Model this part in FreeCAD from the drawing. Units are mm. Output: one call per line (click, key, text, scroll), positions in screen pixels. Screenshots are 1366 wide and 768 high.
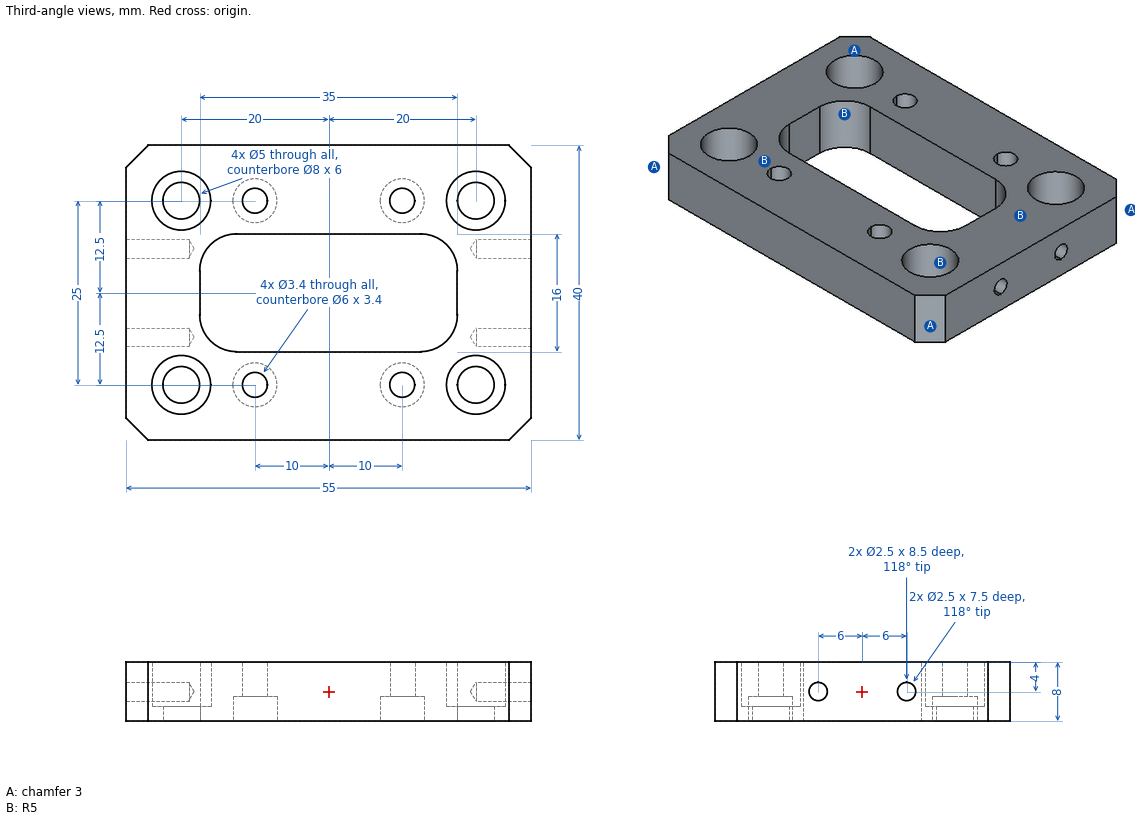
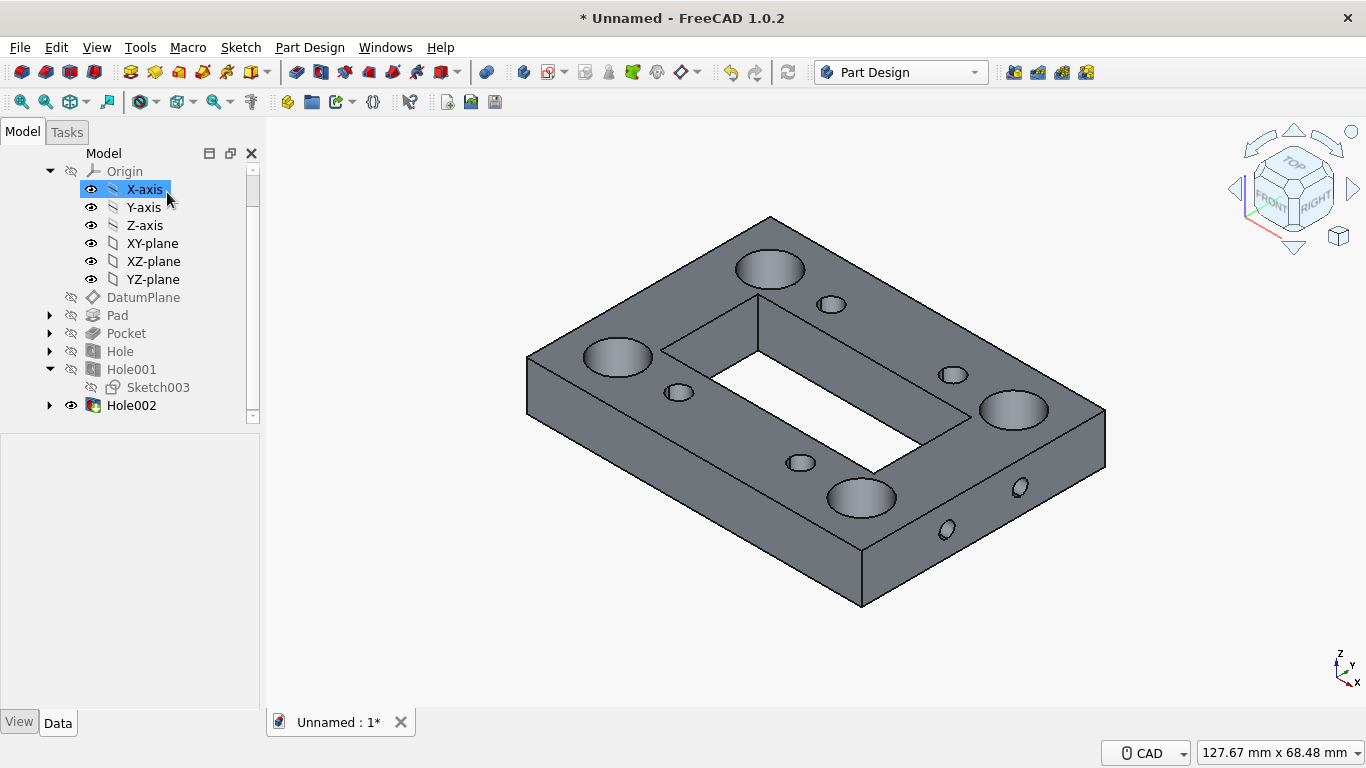
key(6)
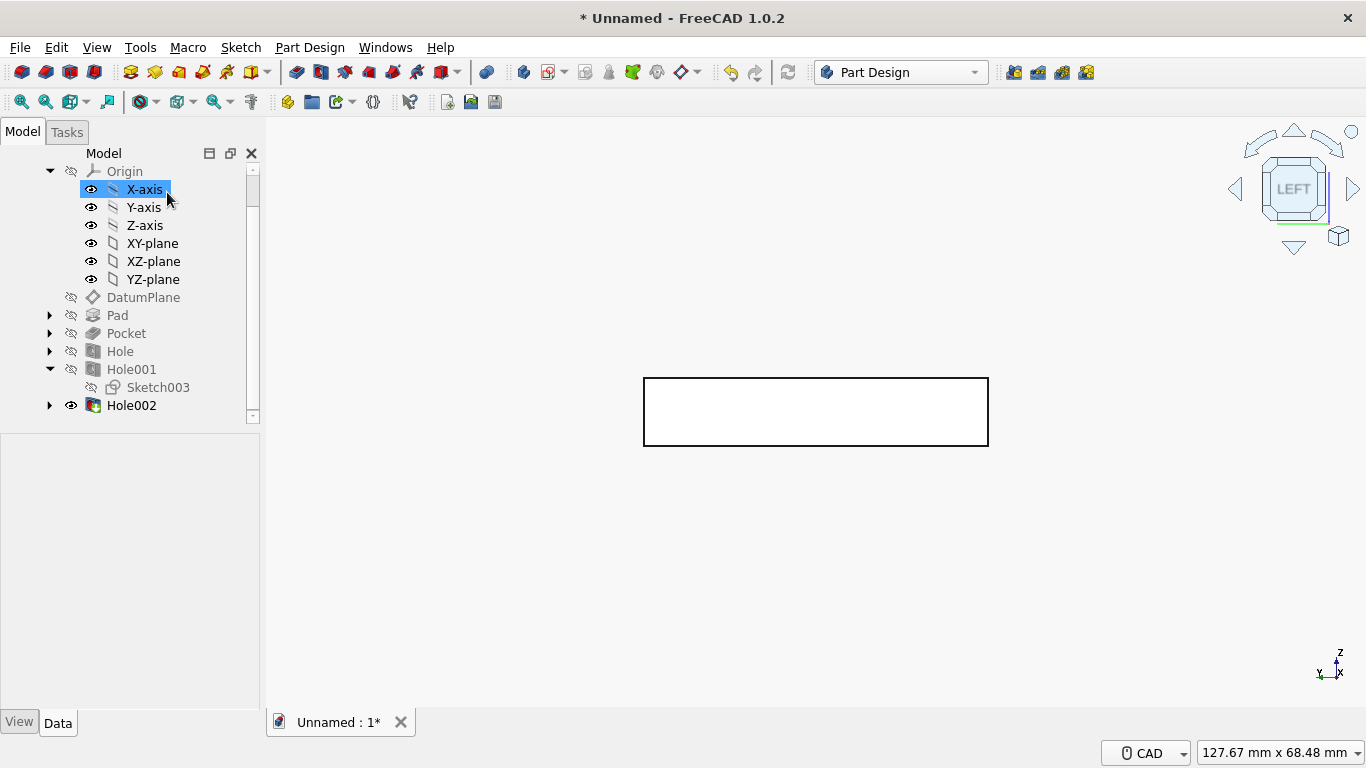
click(22, 102)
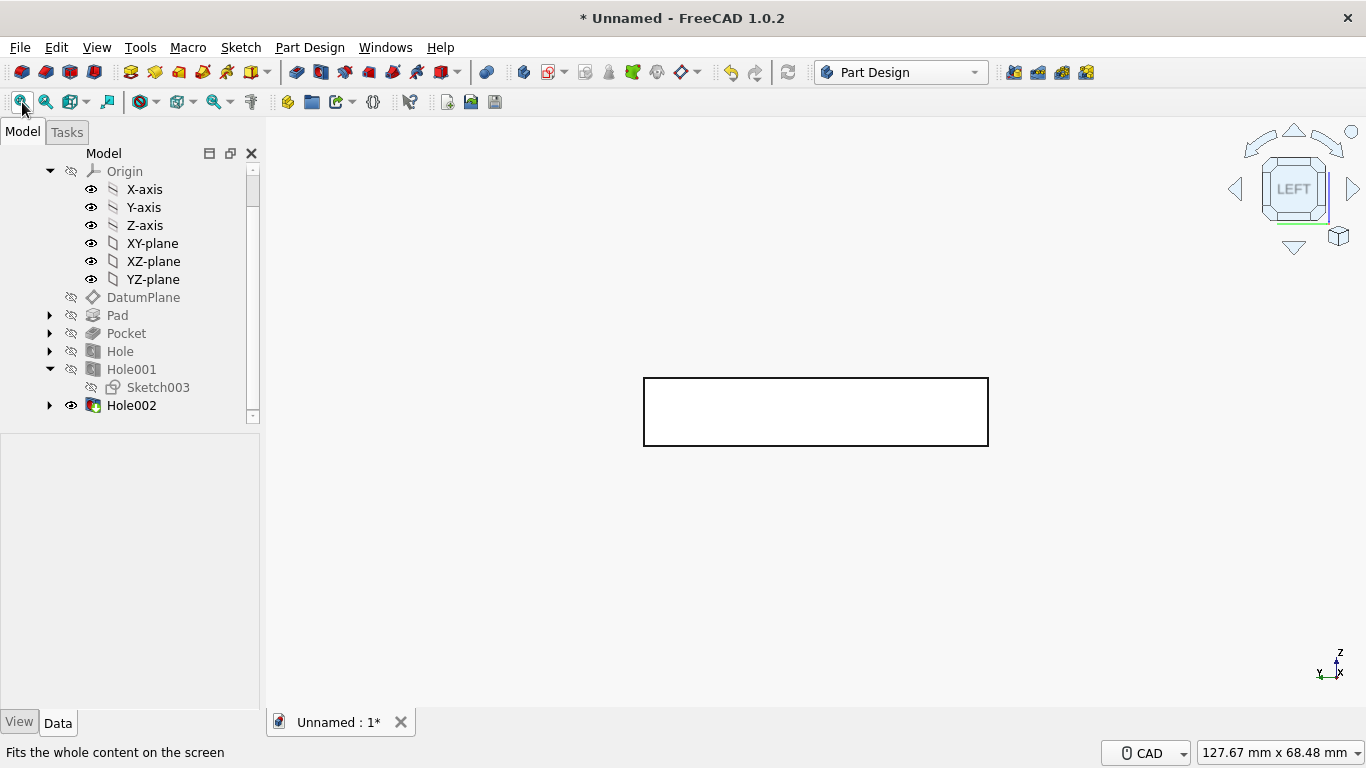
click(718, 411)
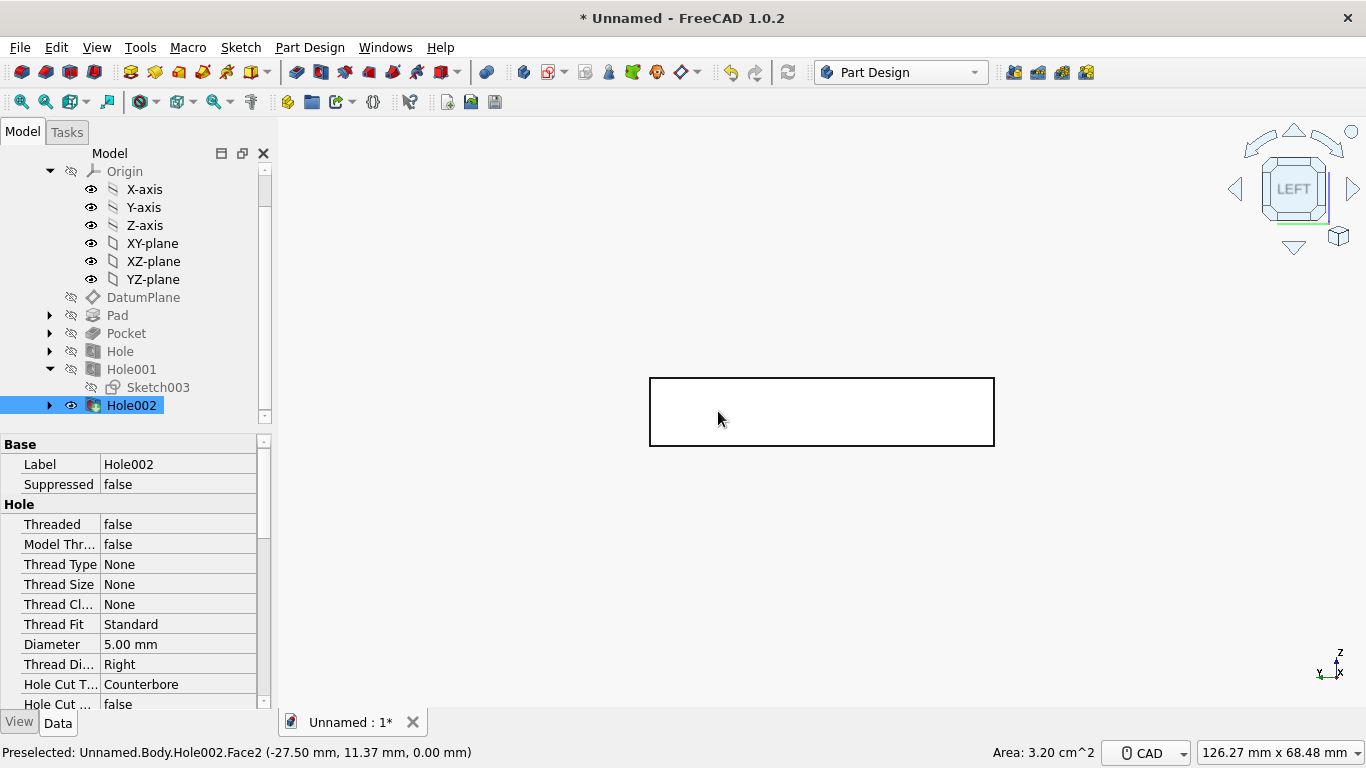
click(548, 72)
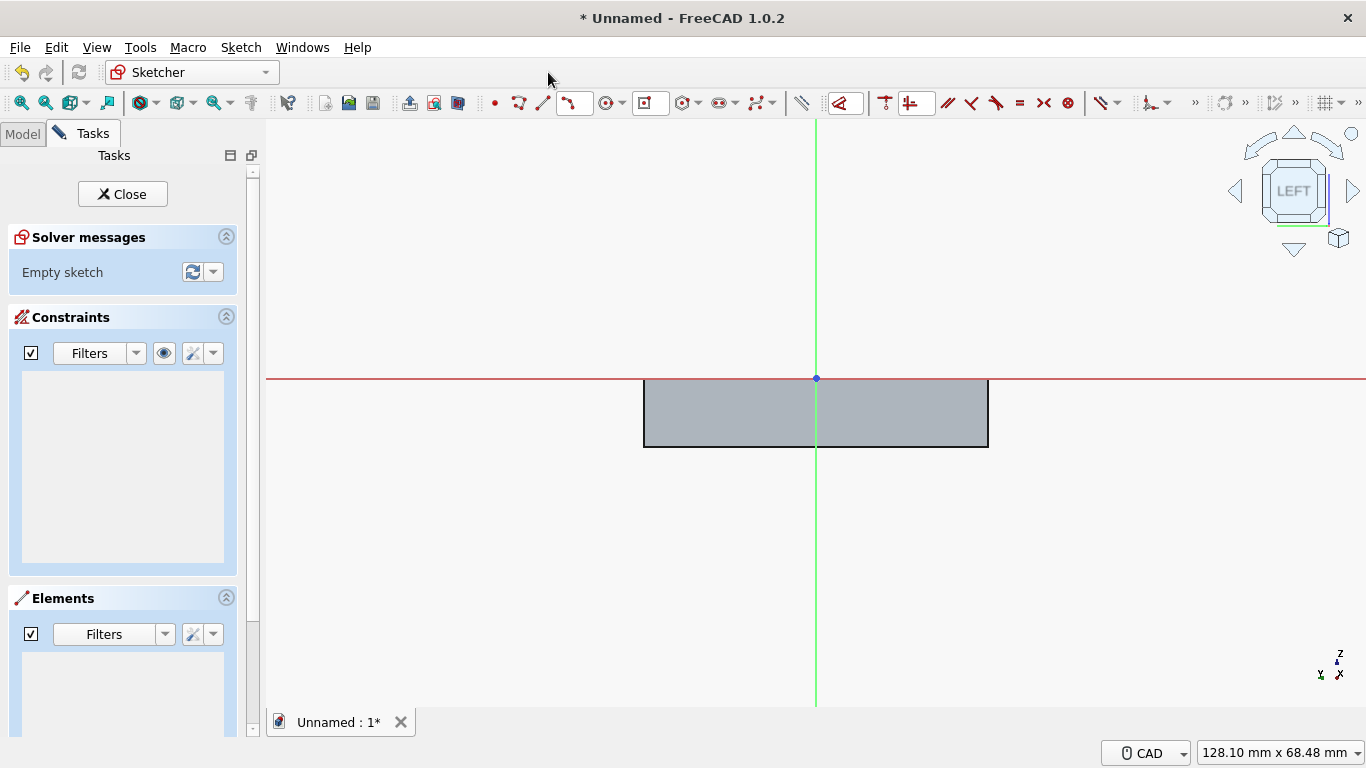
scroll(833, 398, up, 8)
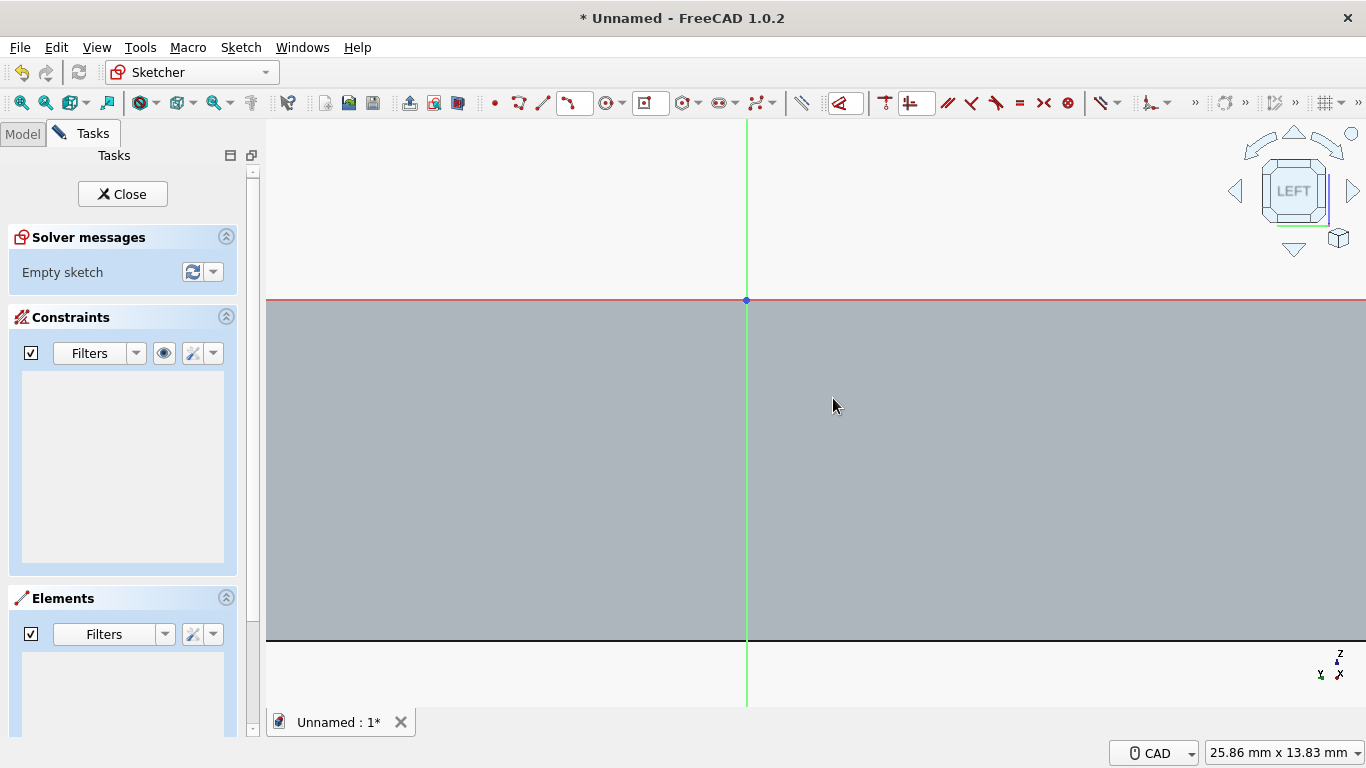
click(606, 104)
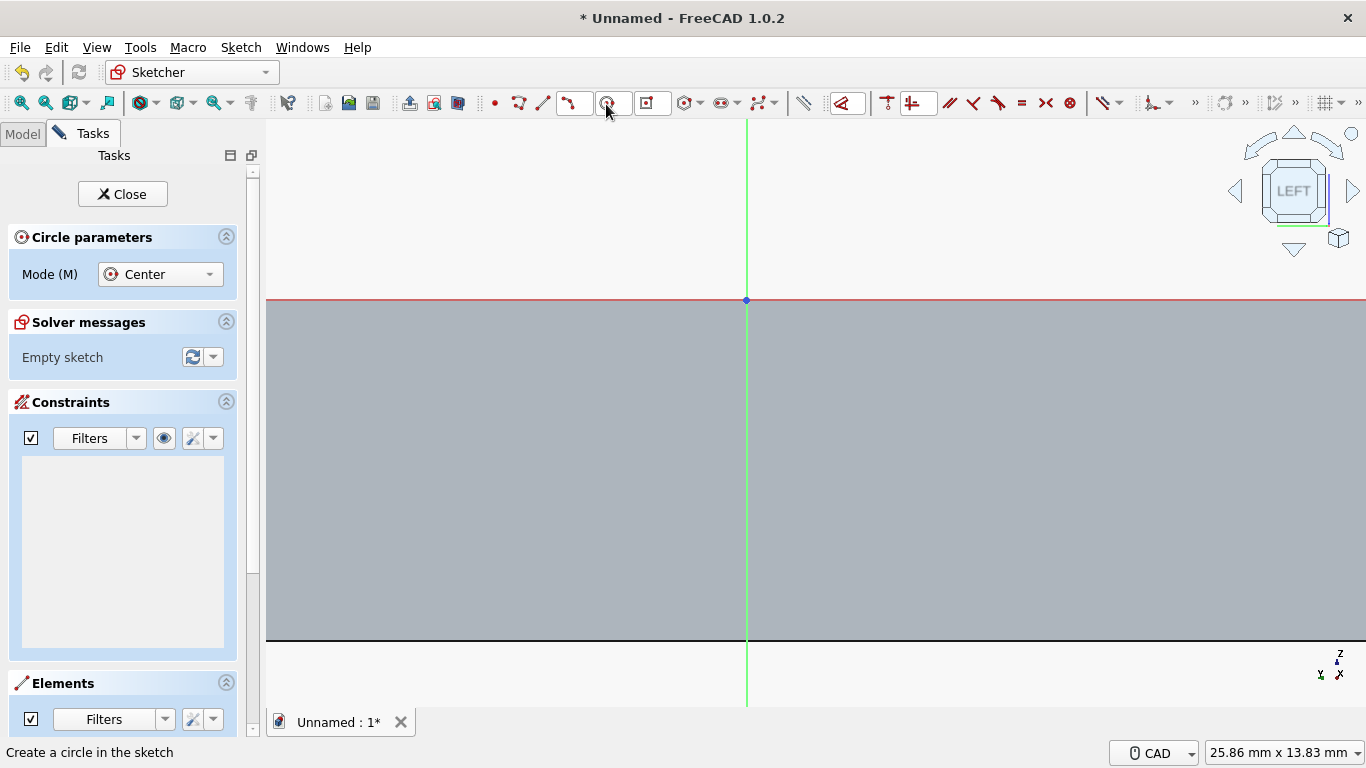
click(492, 470)
move(529, 433)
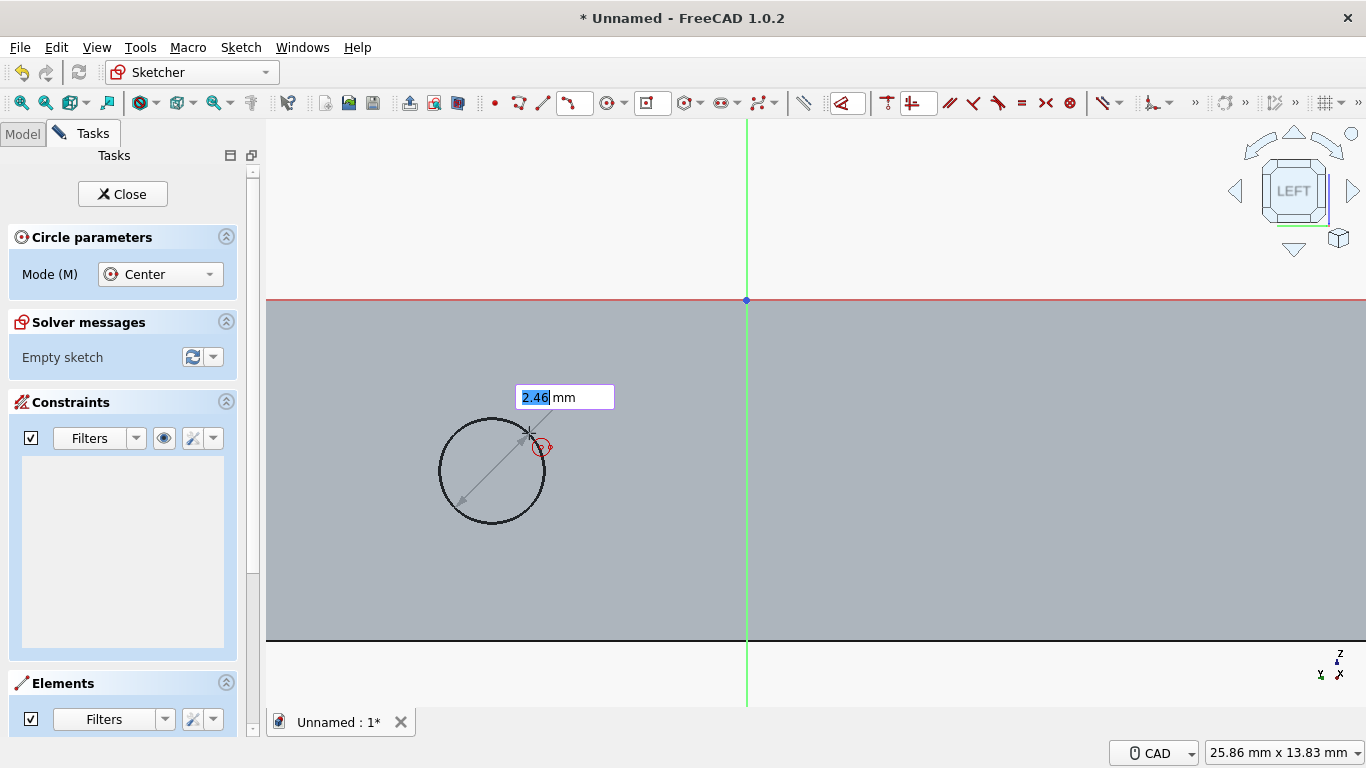
text(2.5)
key(Return)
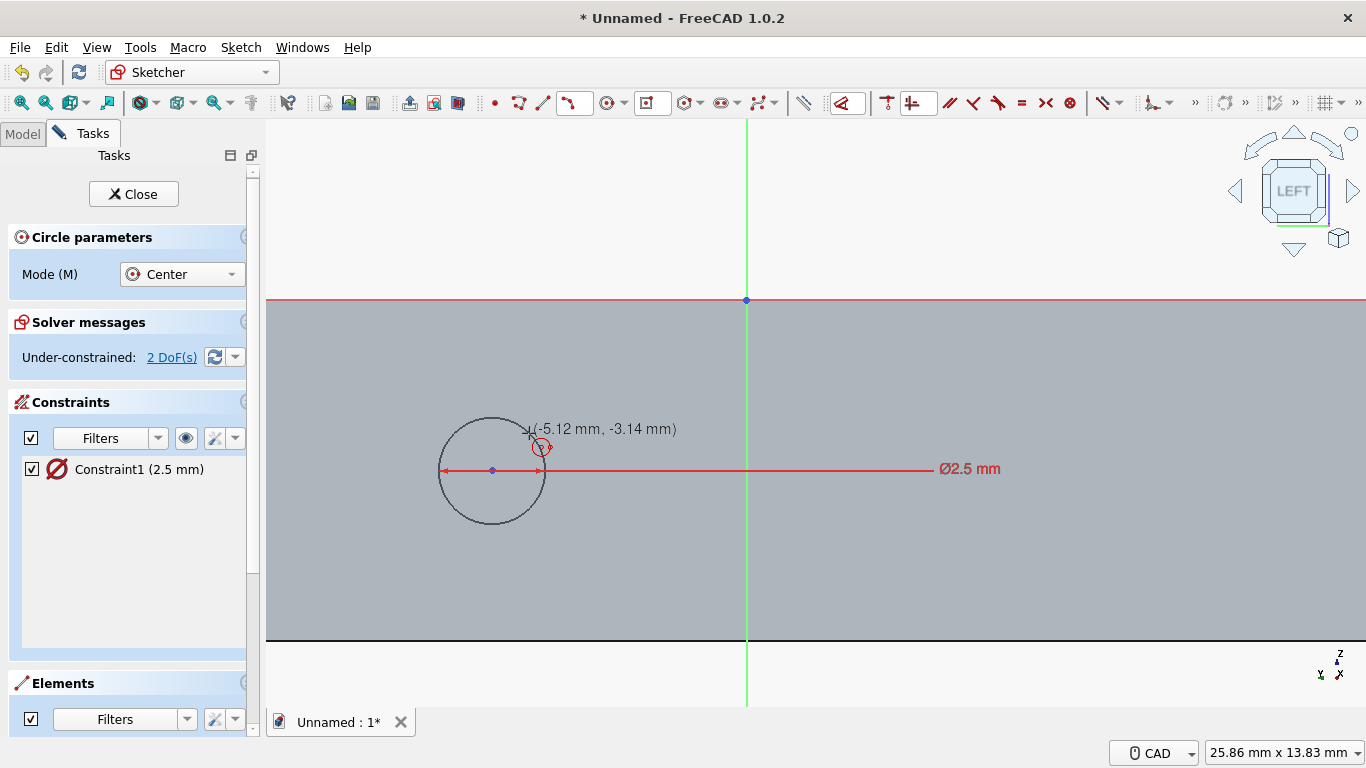
click(1002, 470)
move(1040, 433)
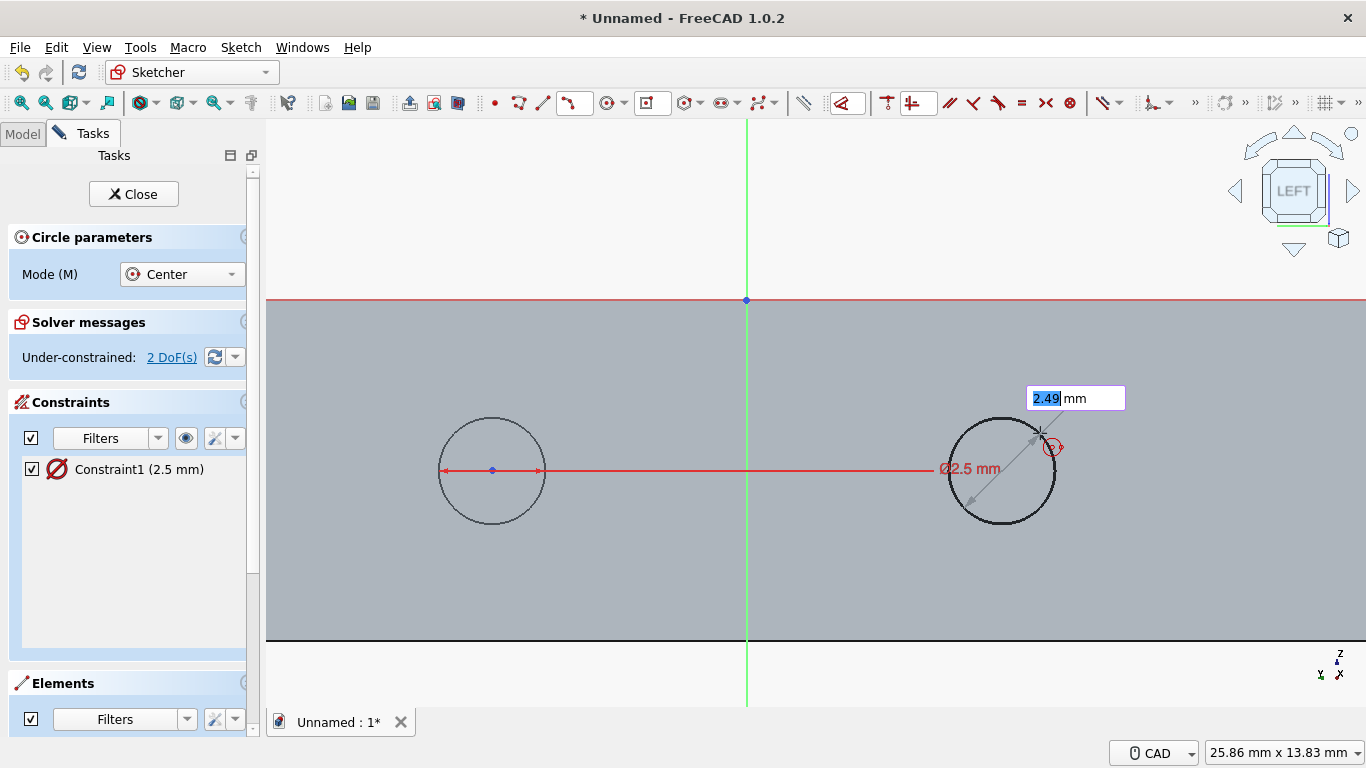
text(2.5)
key(Return)
key(Escape)